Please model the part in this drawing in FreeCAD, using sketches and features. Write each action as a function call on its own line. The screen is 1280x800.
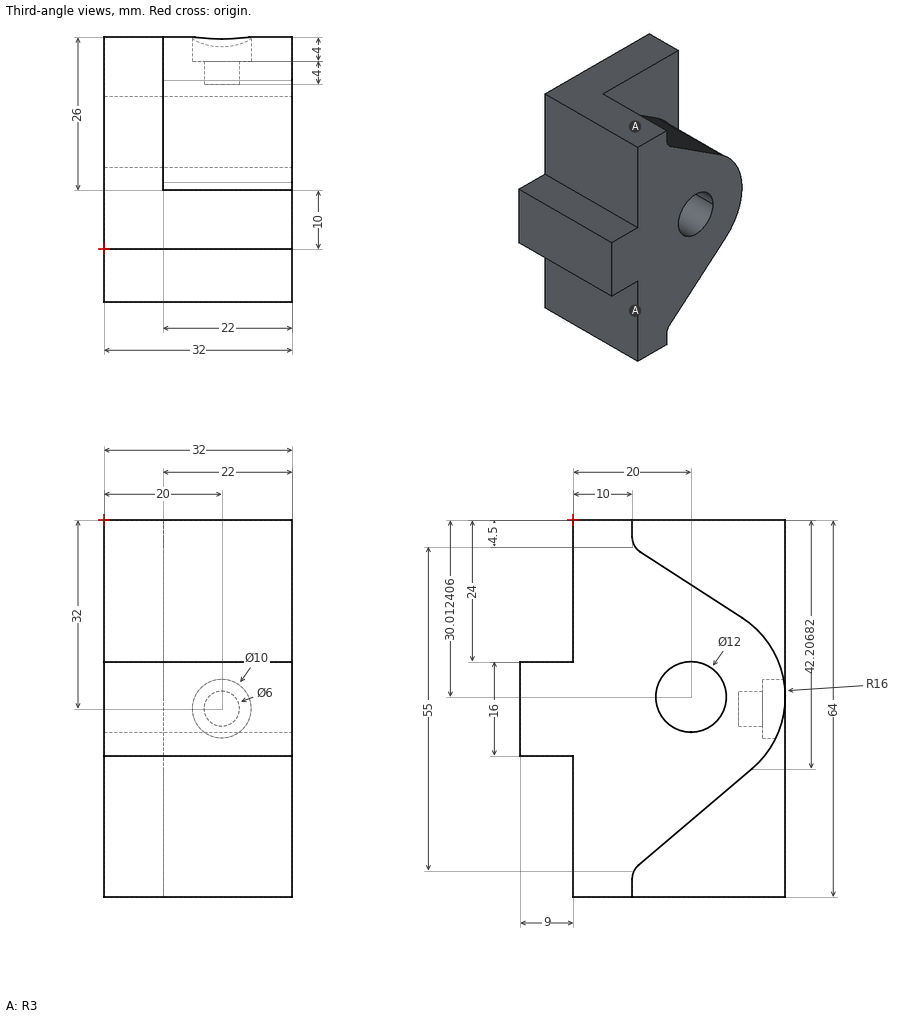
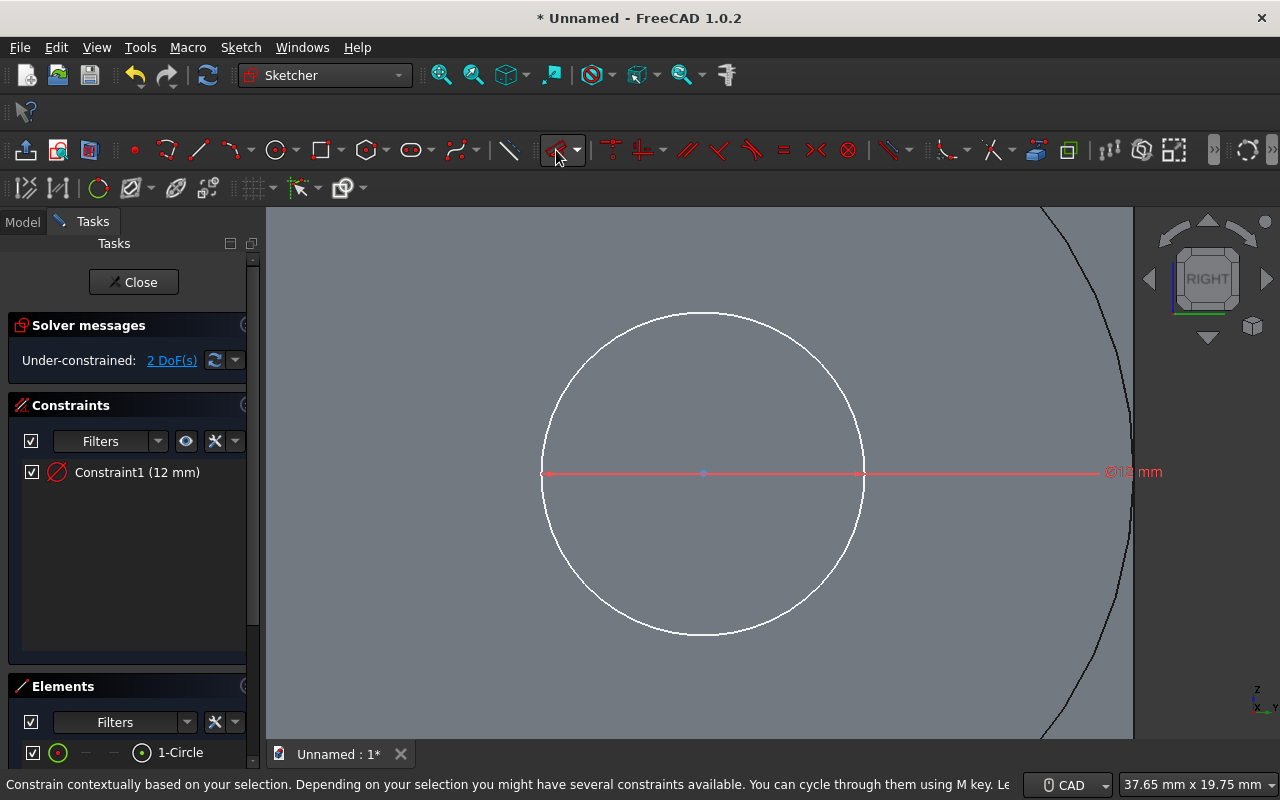
click(703, 474)
click(499, 508)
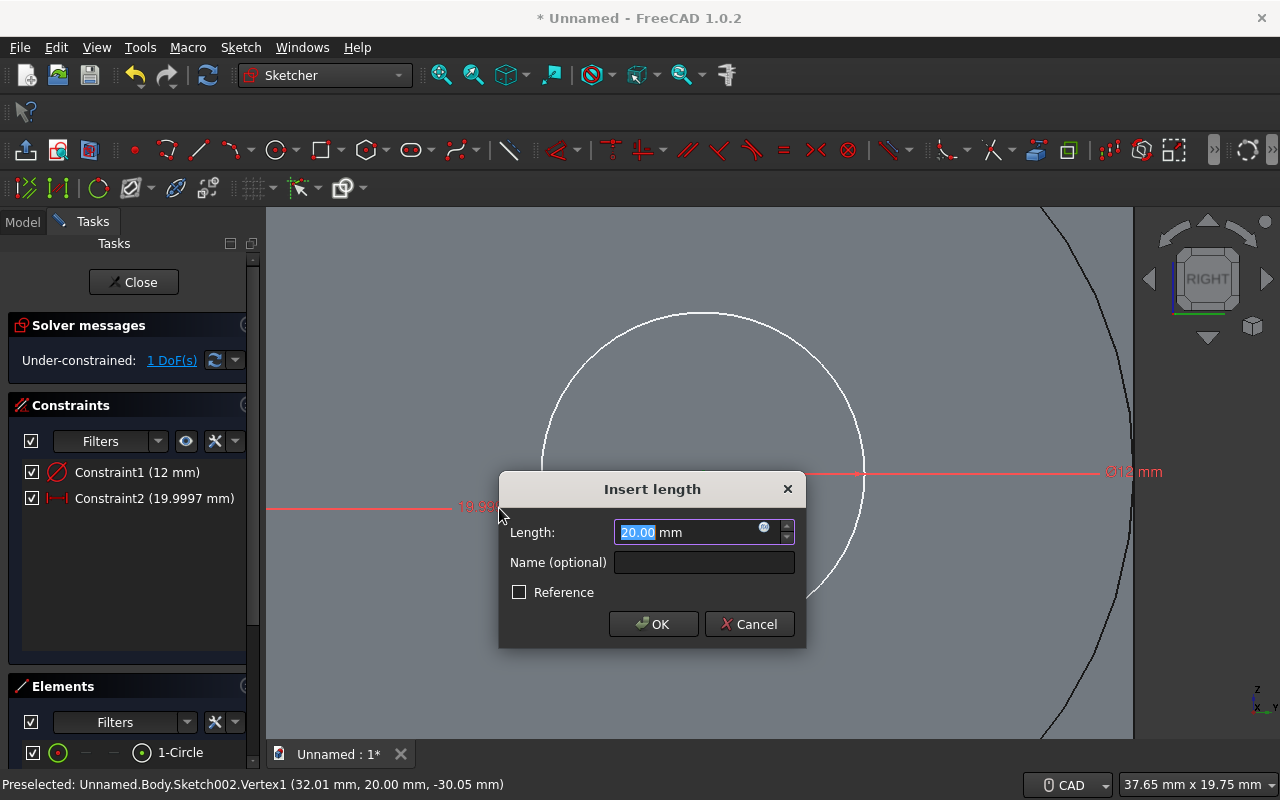
text(20)
key(Return)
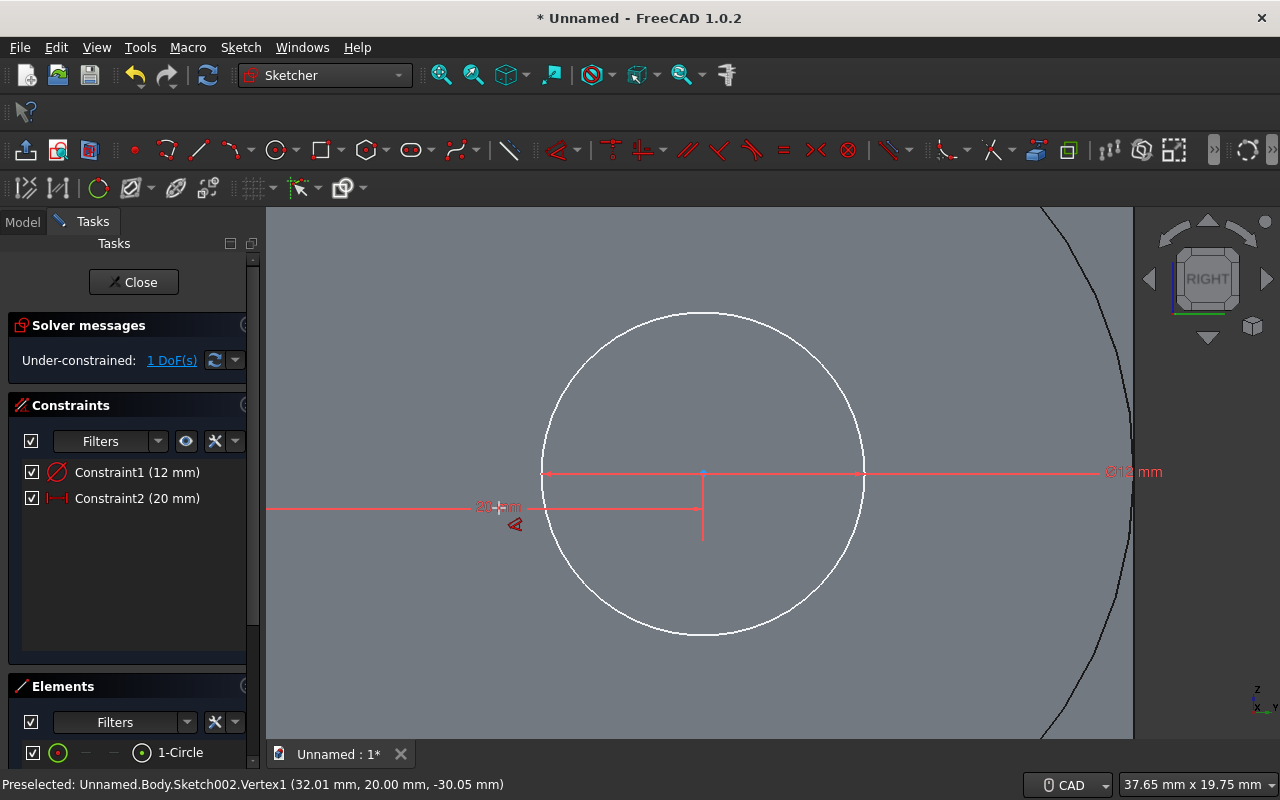
click(703, 474)
click(737, 354)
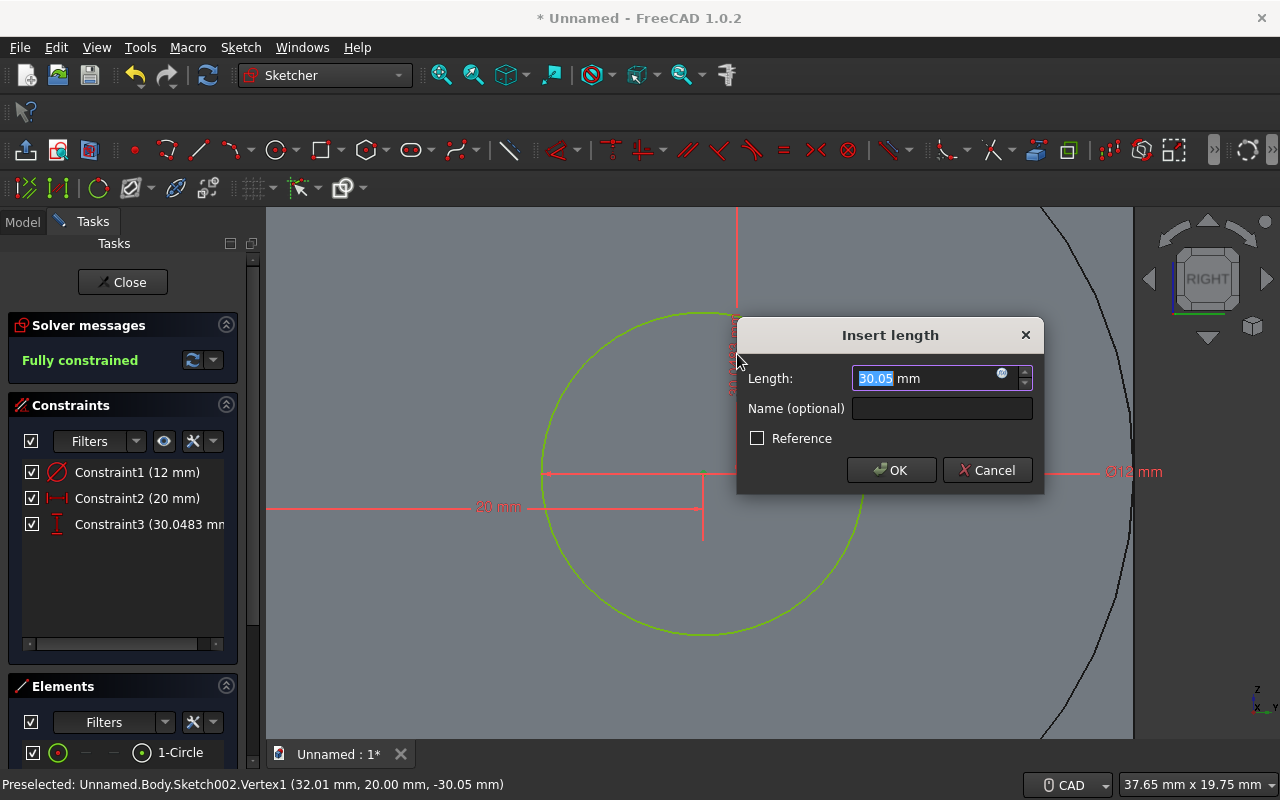
text(30.012406)
key(Return)
key(Escape)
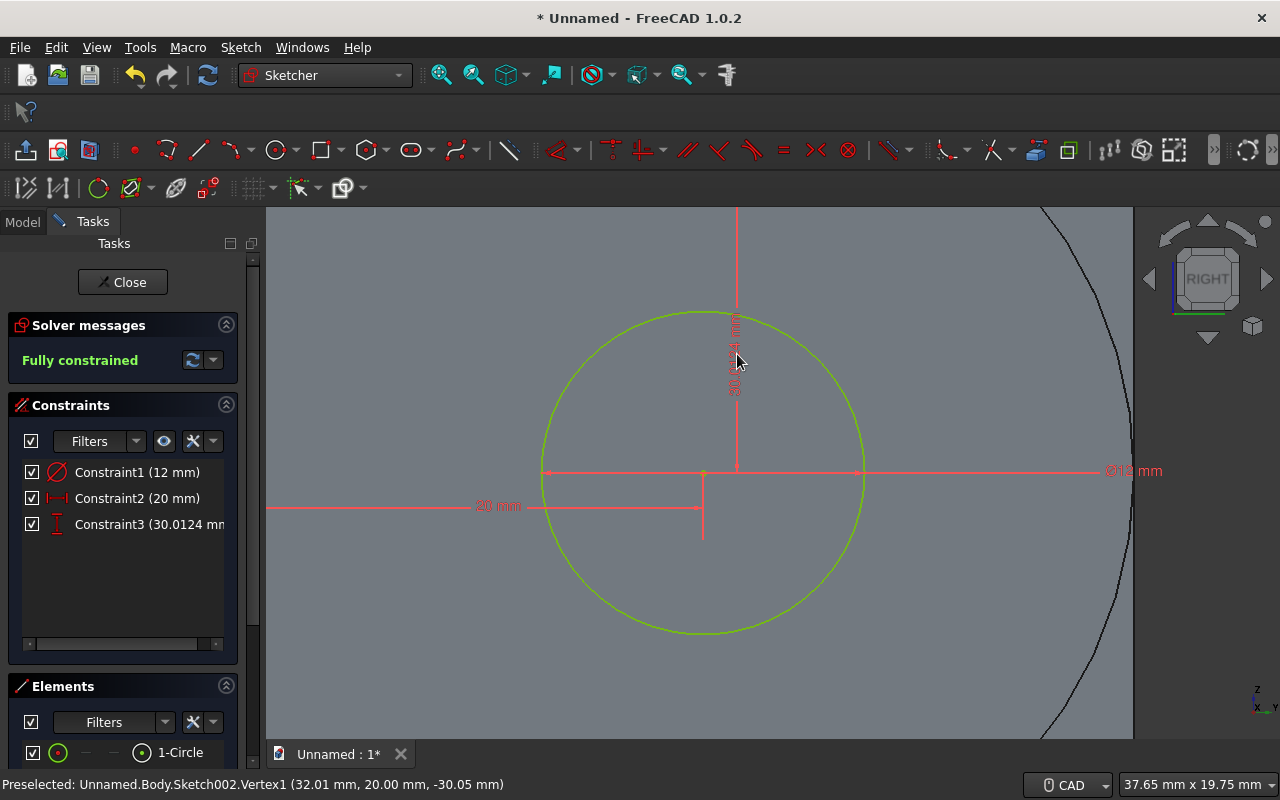
click(123, 282)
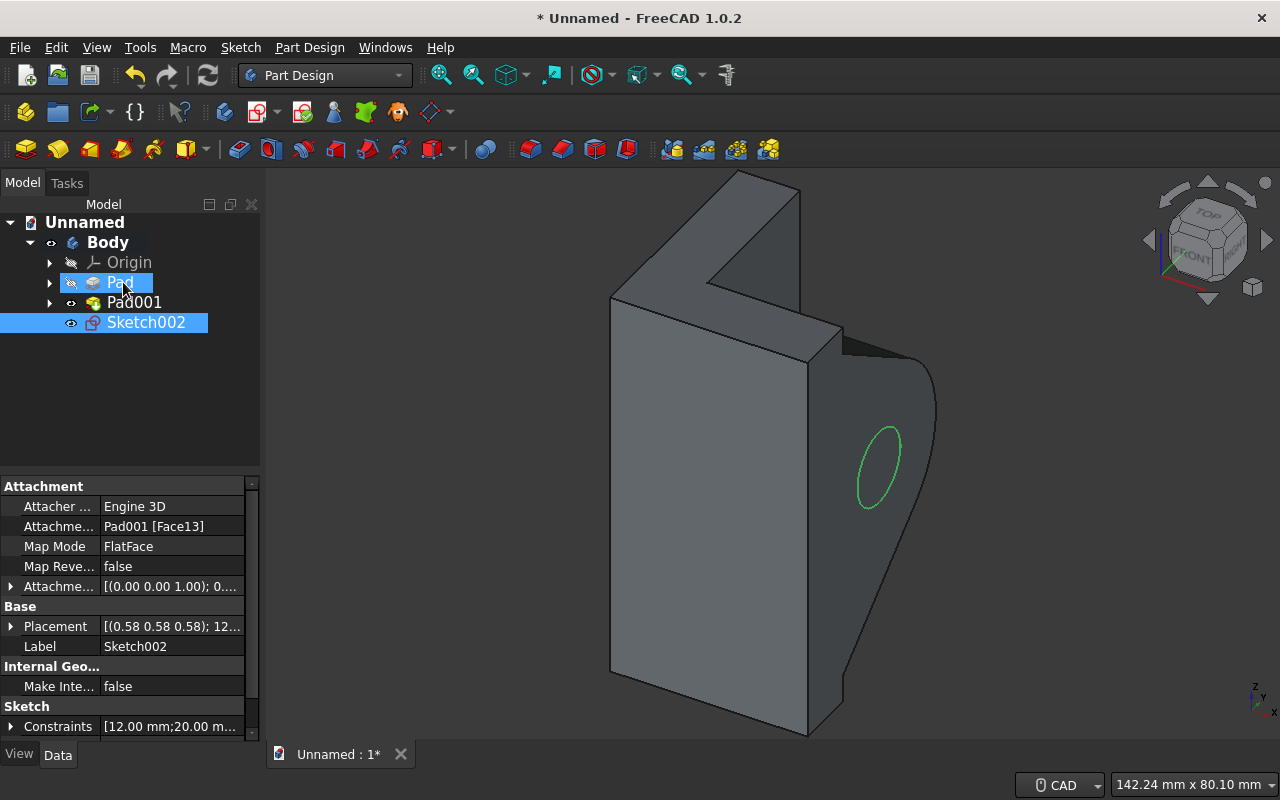
click(240, 150)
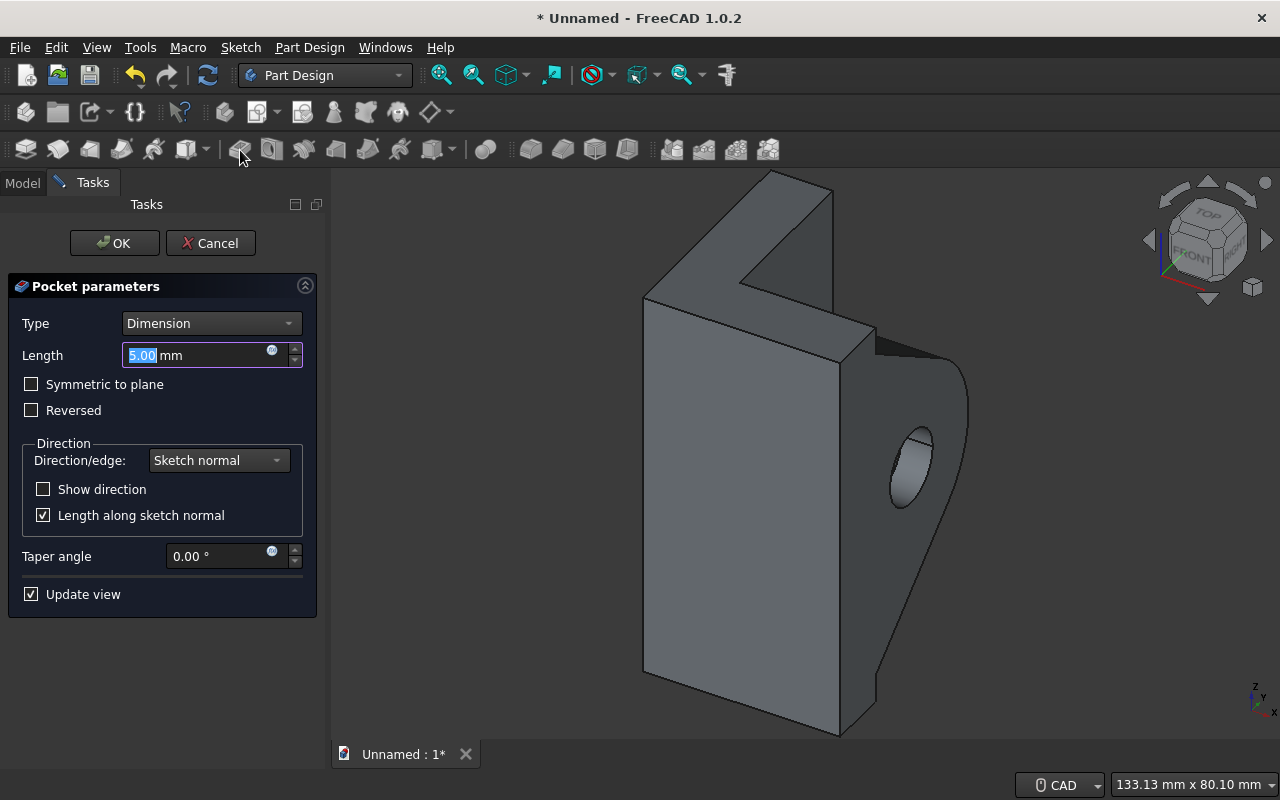
text(32)
key(Tab)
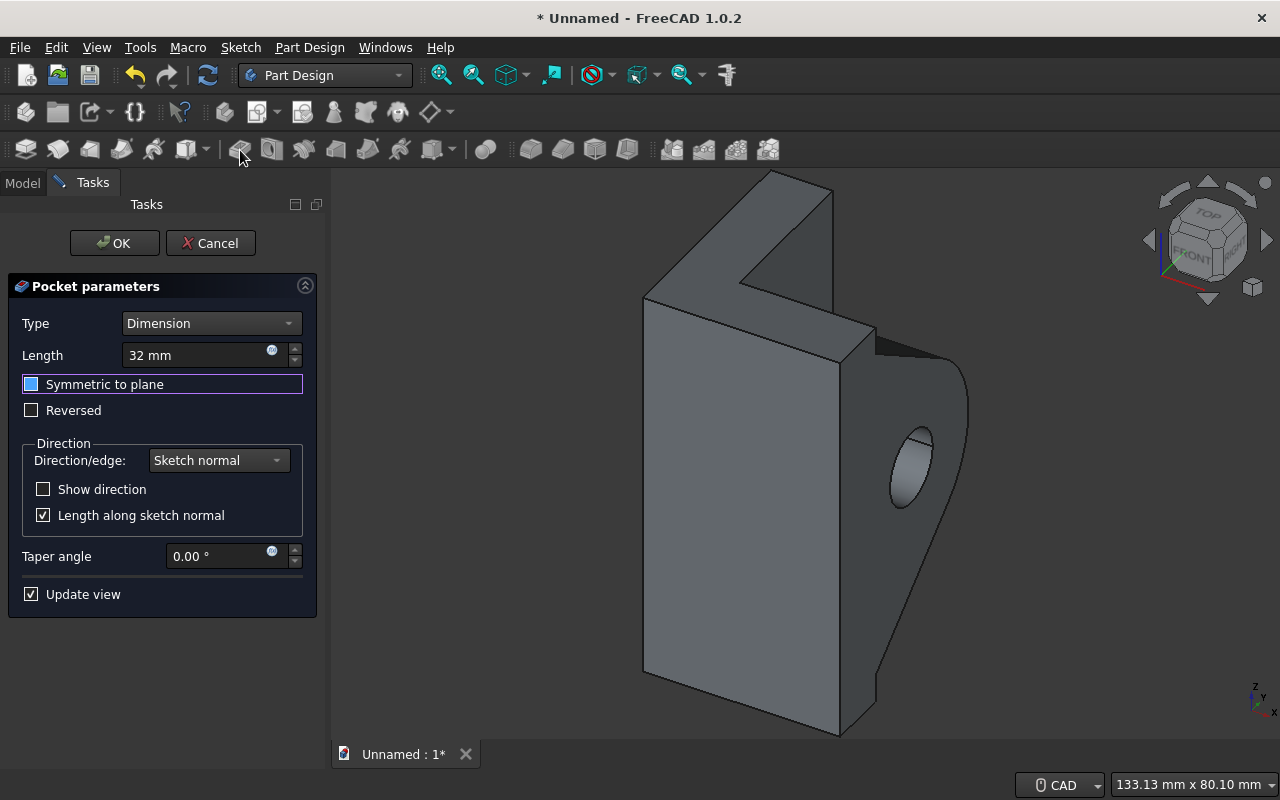
click(115, 243)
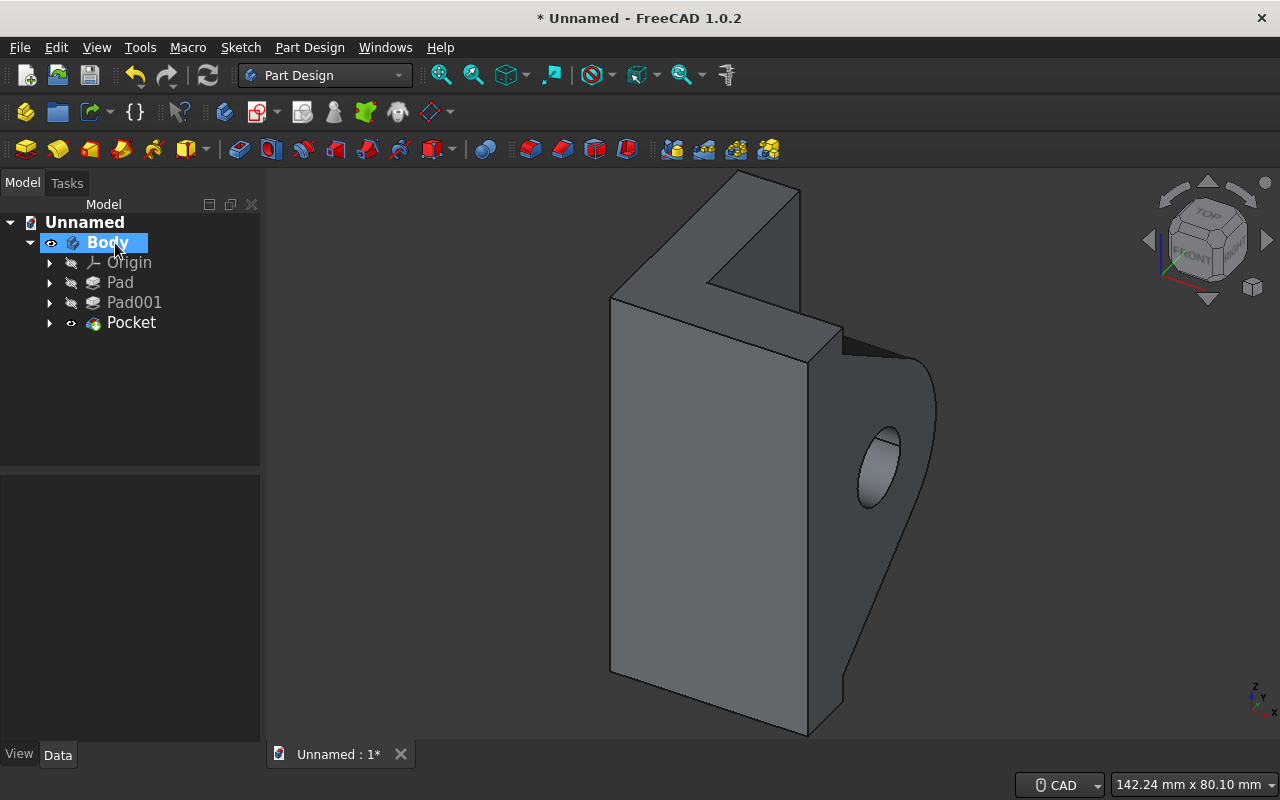
click(835, 415)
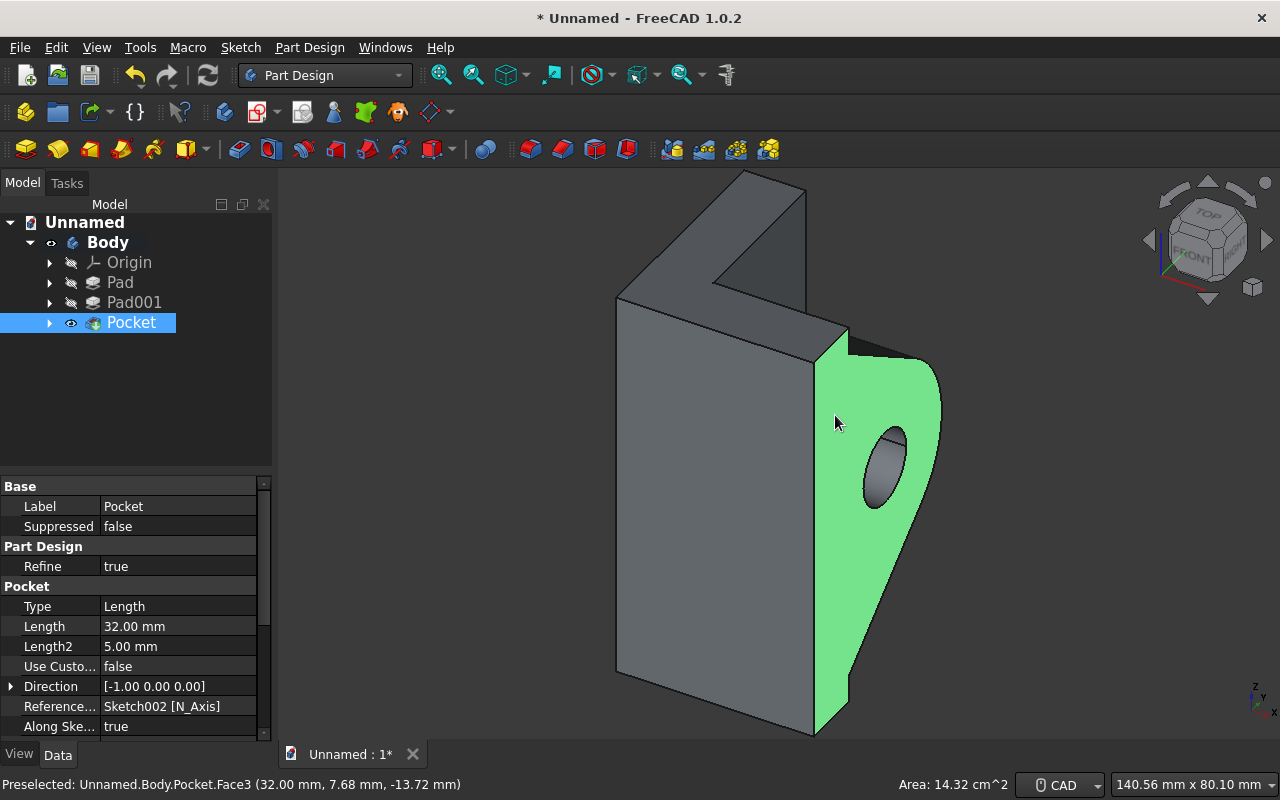
click(258, 112)